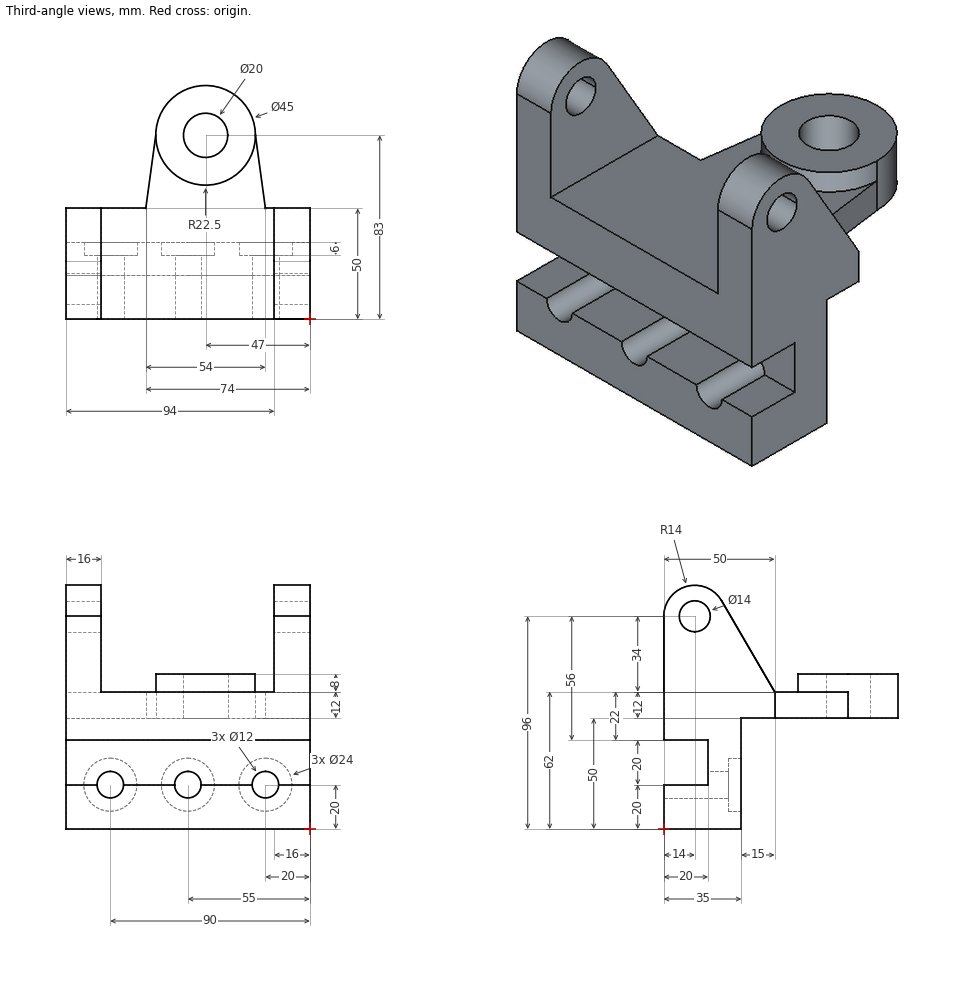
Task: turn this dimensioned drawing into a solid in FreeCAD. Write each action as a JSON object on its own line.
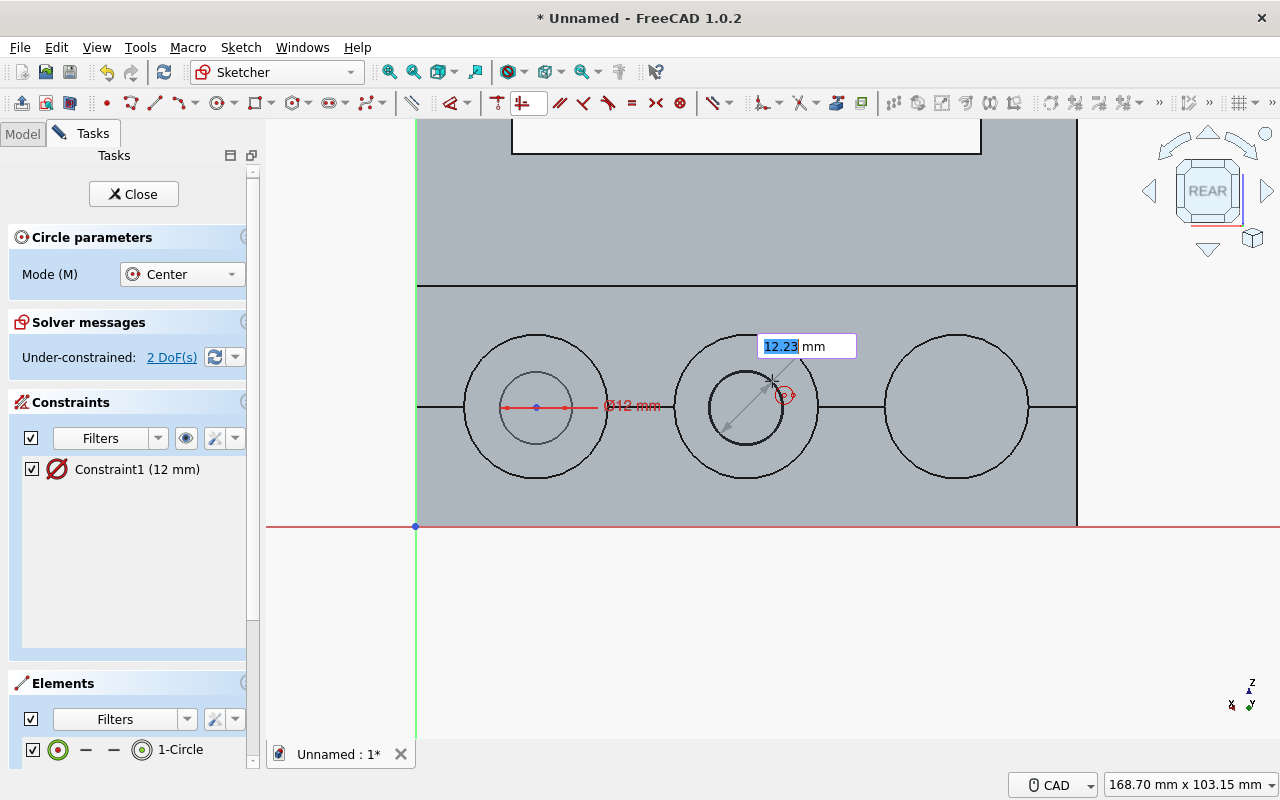
{"action": "type", "text": "12"}
{"action": "key", "text": "Return"}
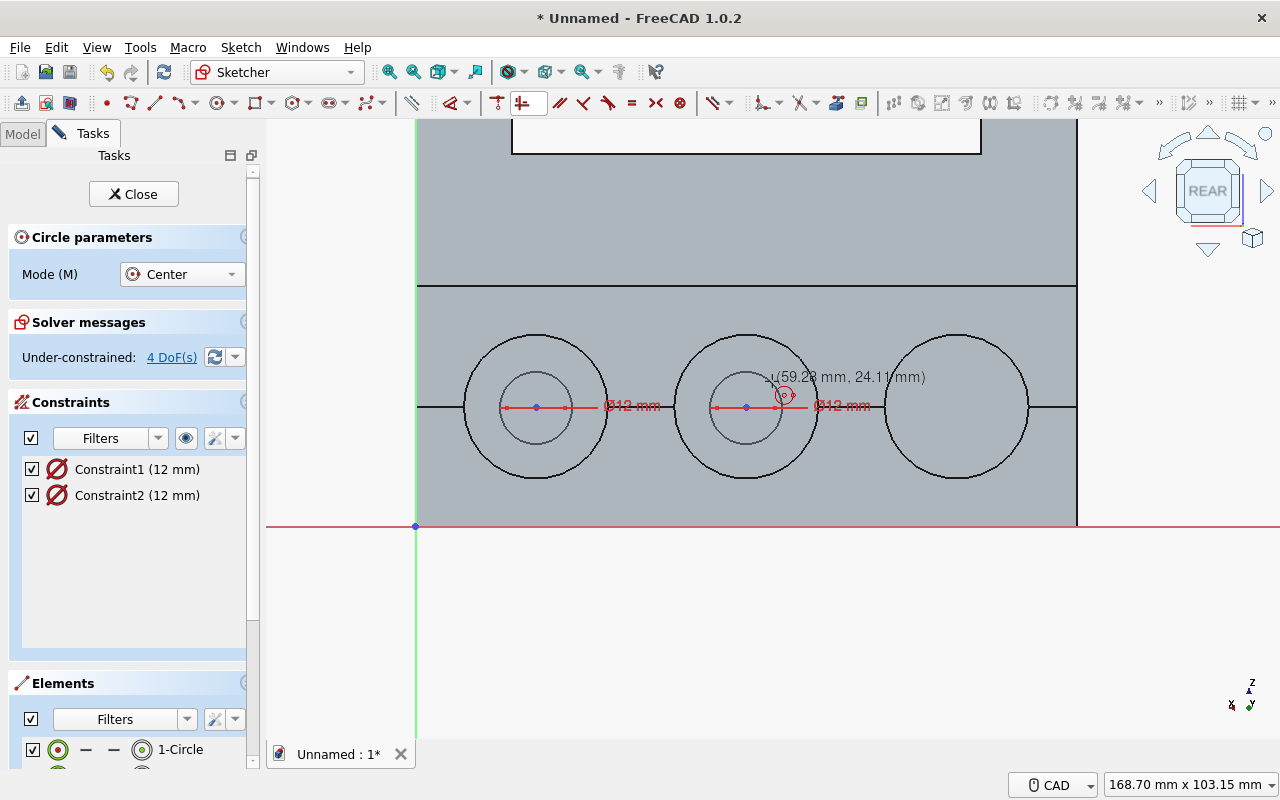
{"action": "left_click", "coordinate": [957, 407]}
{"action": "mouse_move", "coordinate": [982, 381]}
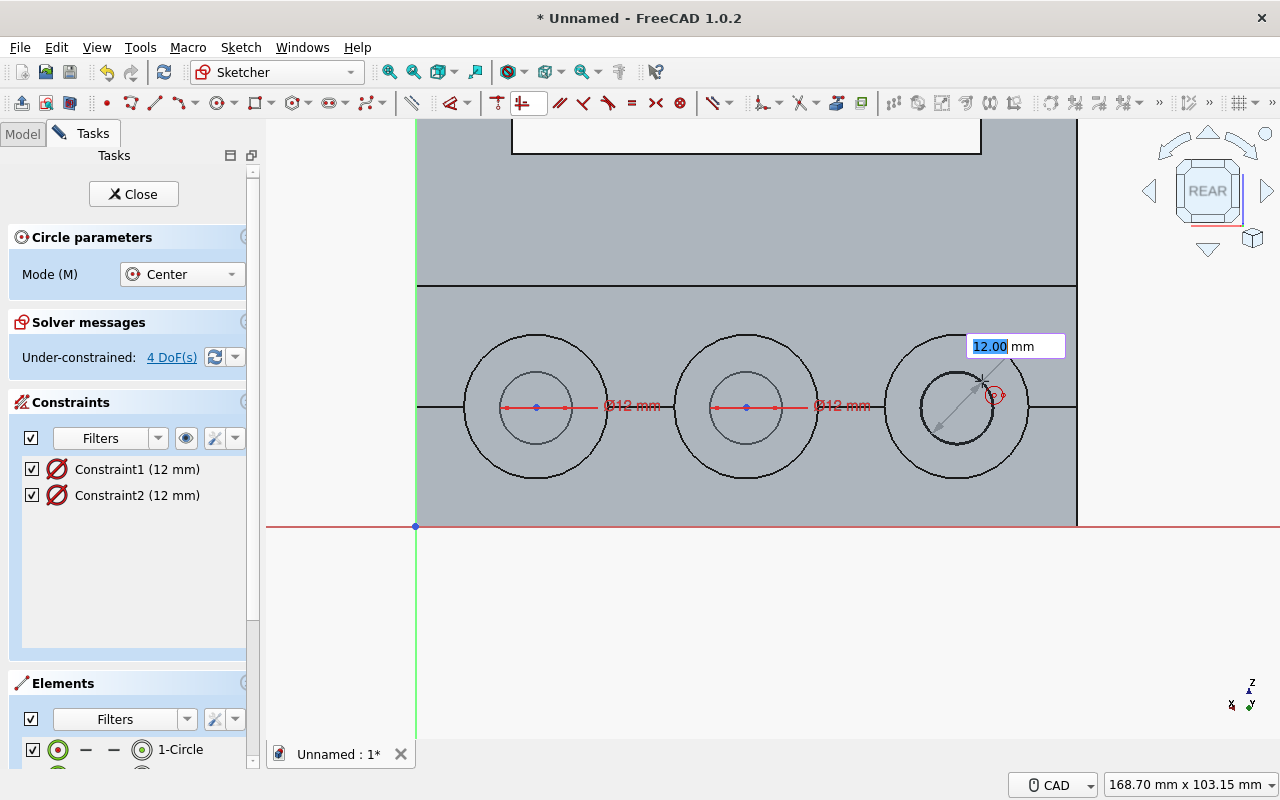
{"action": "type", "text": "12"}
{"action": "key", "text": "Return"}
{"action": "key", "text": "Escape"}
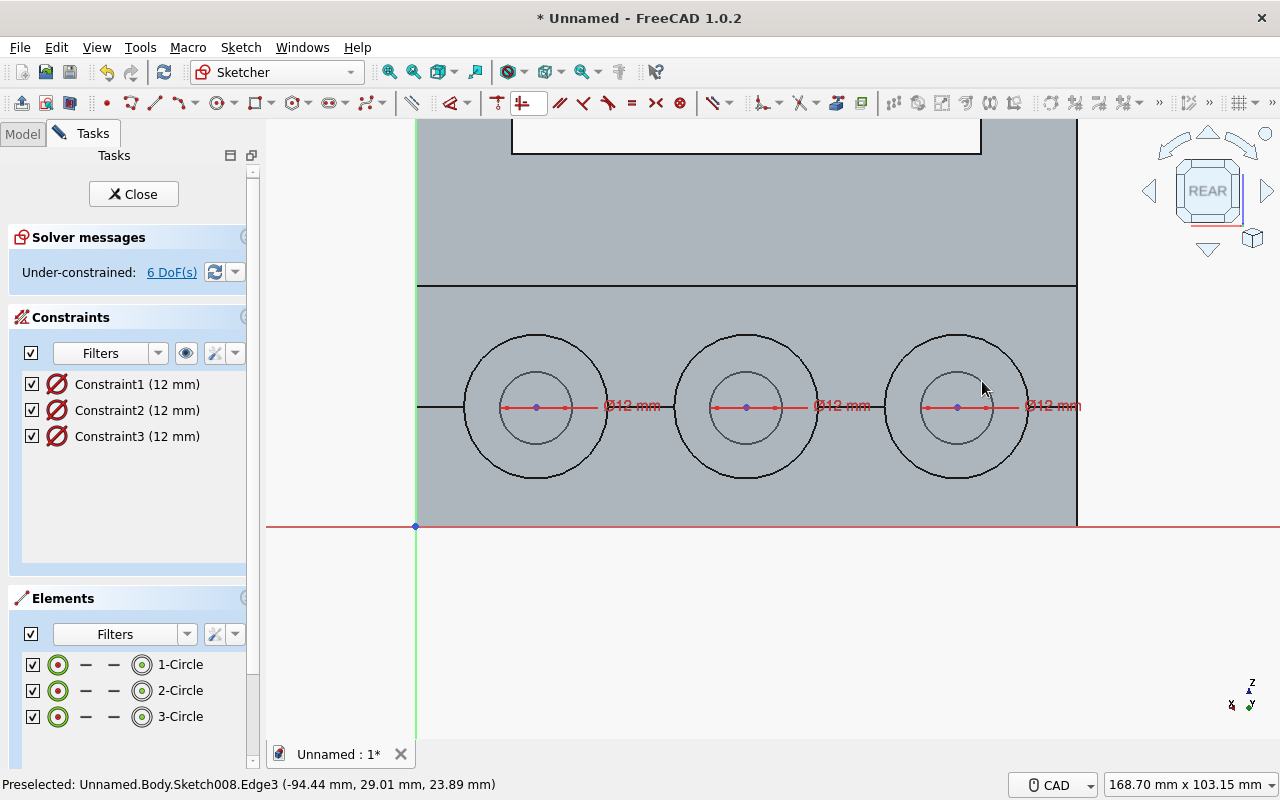
{"action": "left_click", "coordinate": [536, 408]}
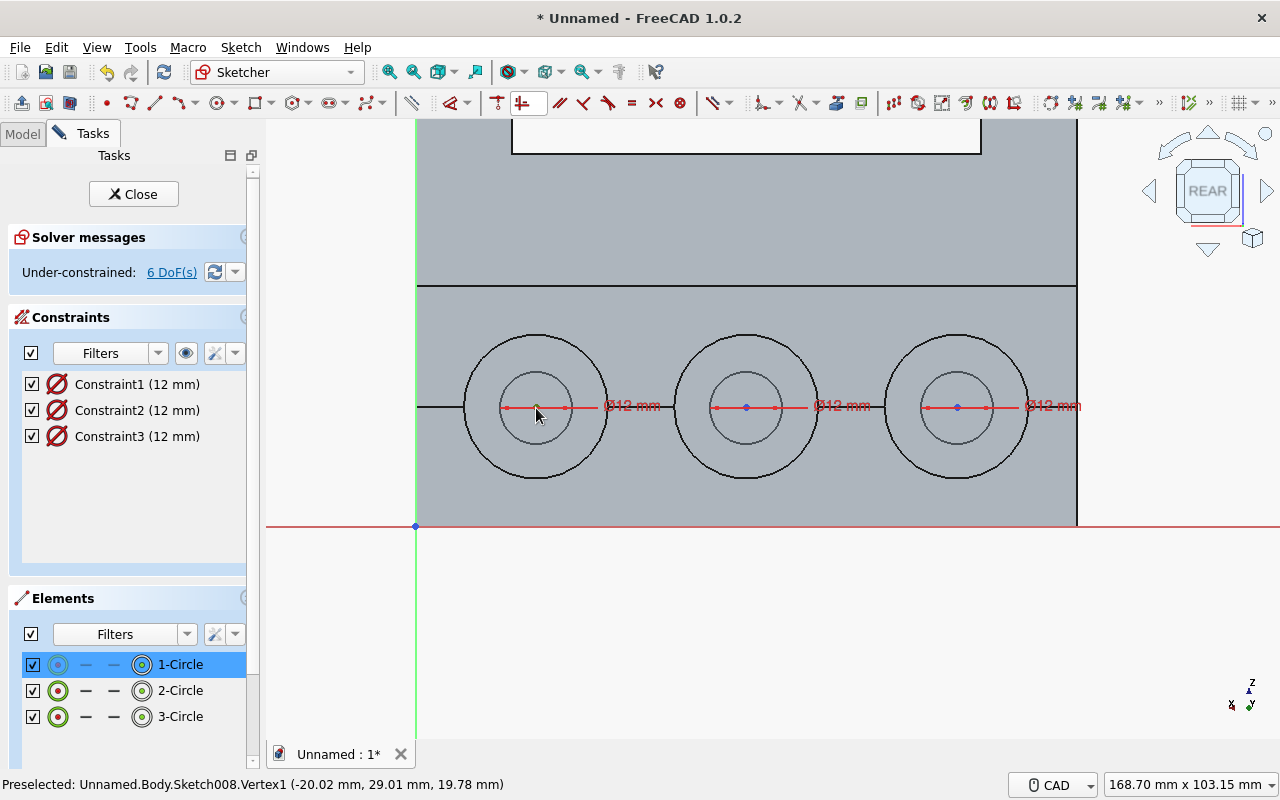
{"action": "left_click", "coordinate": [746, 408]}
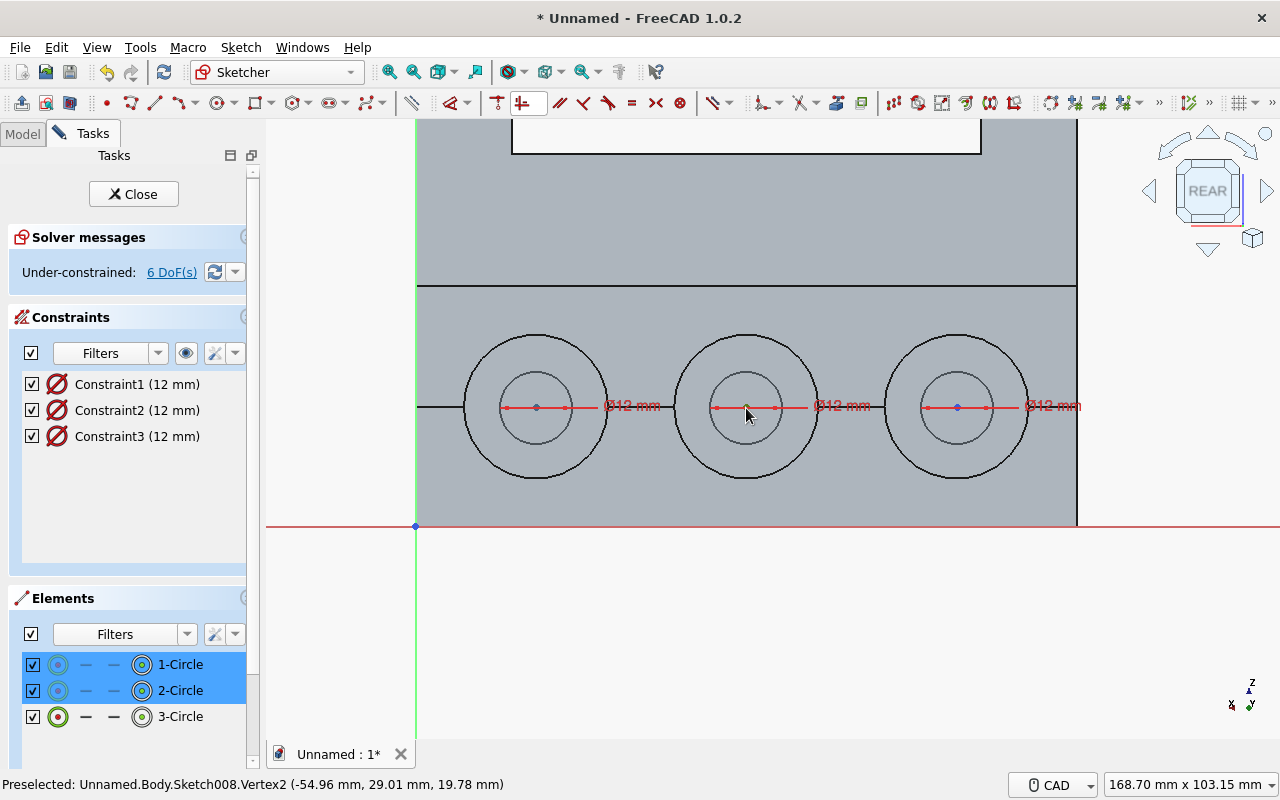
{"action": "left_click", "coordinate": [542, 104]}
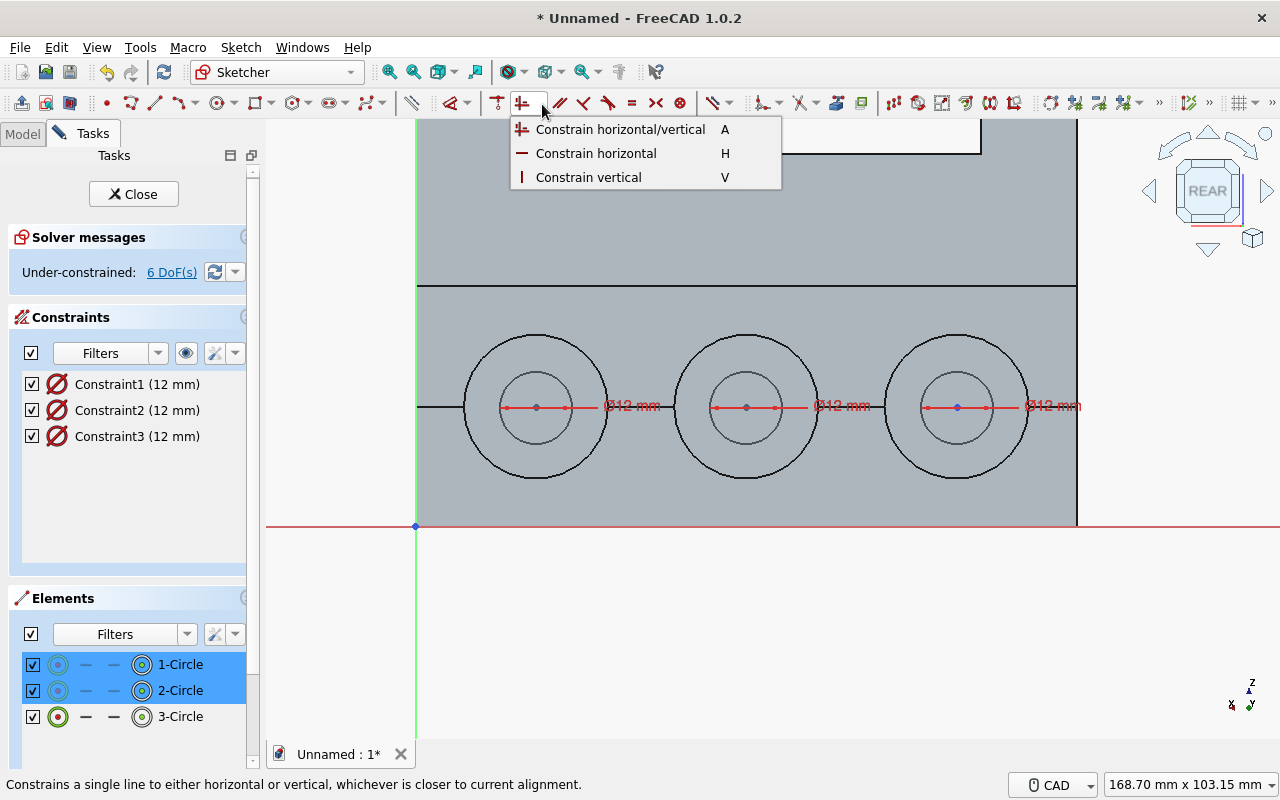
{"action": "left_click", "coordinate": [646, 153]}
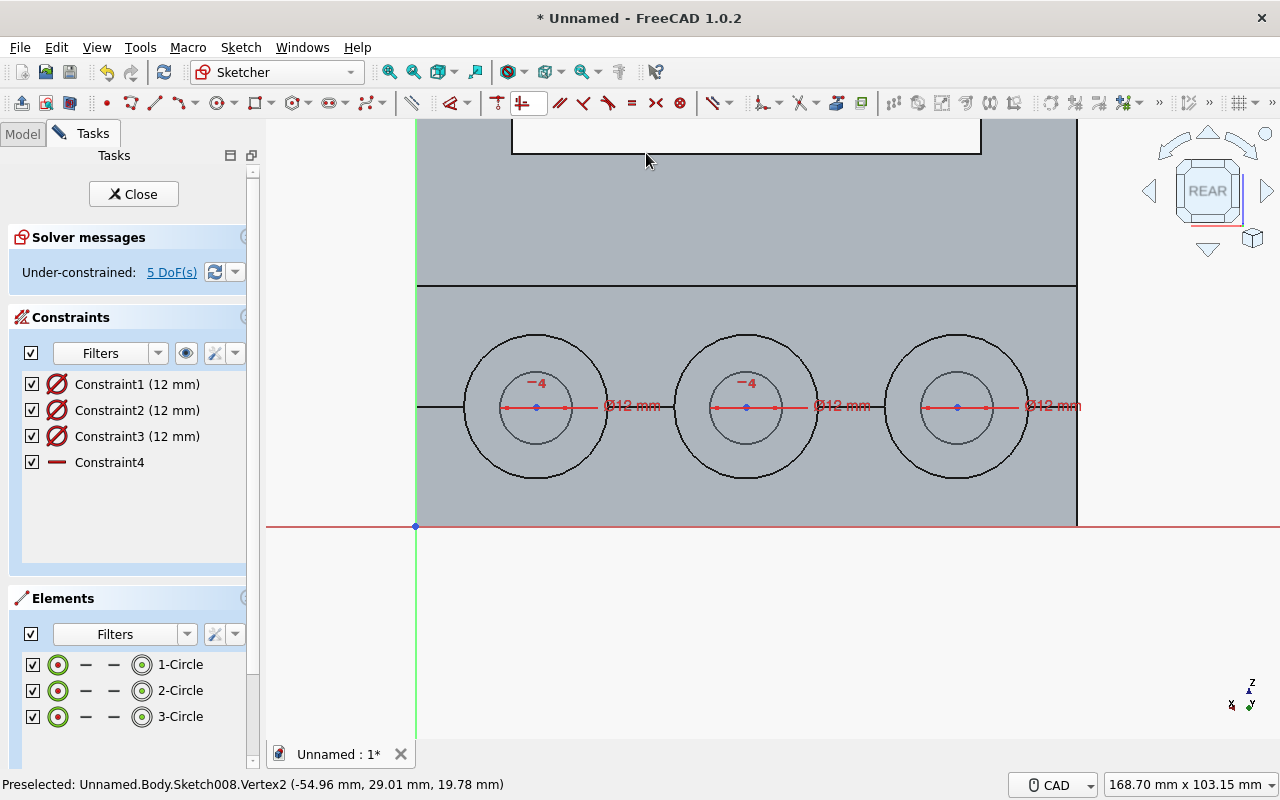
{"action": "left_click", "coordinate": [746, 408]}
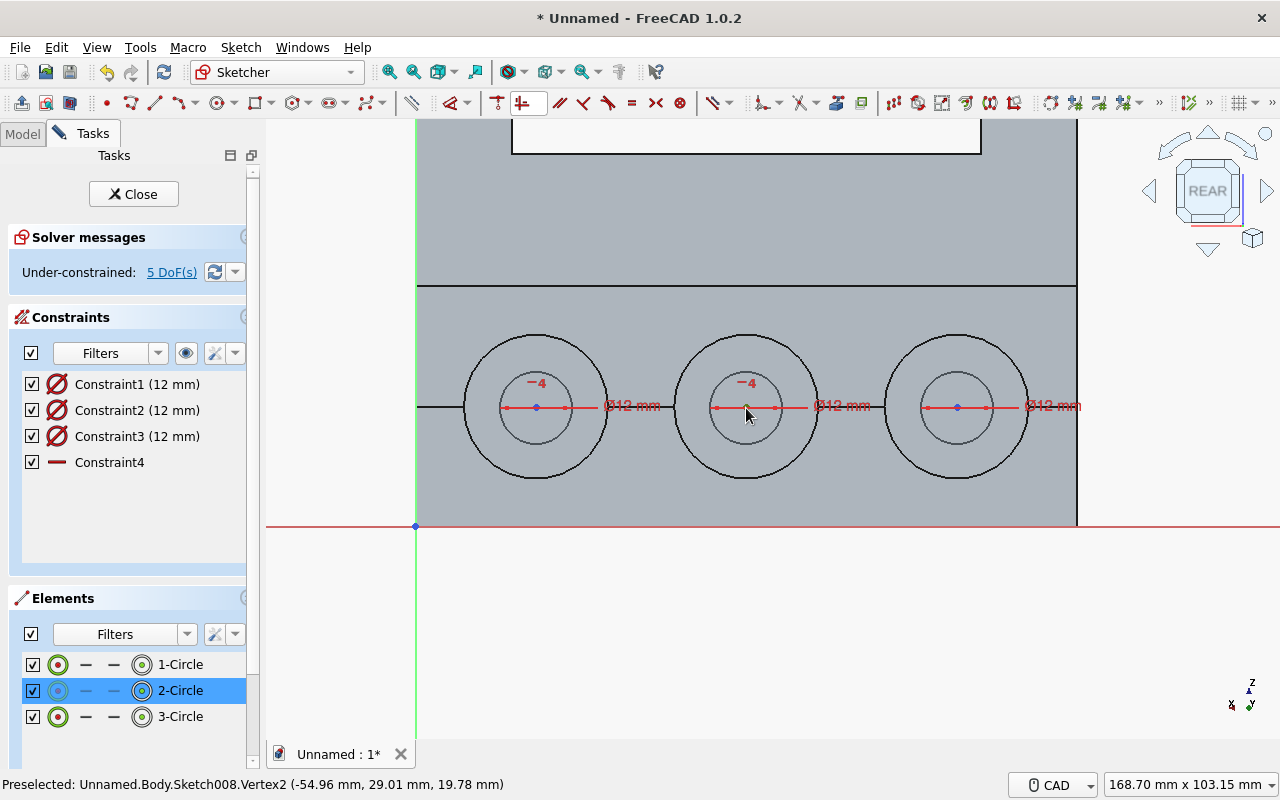
{"action": "left_click", "coordinate": [957, 408]}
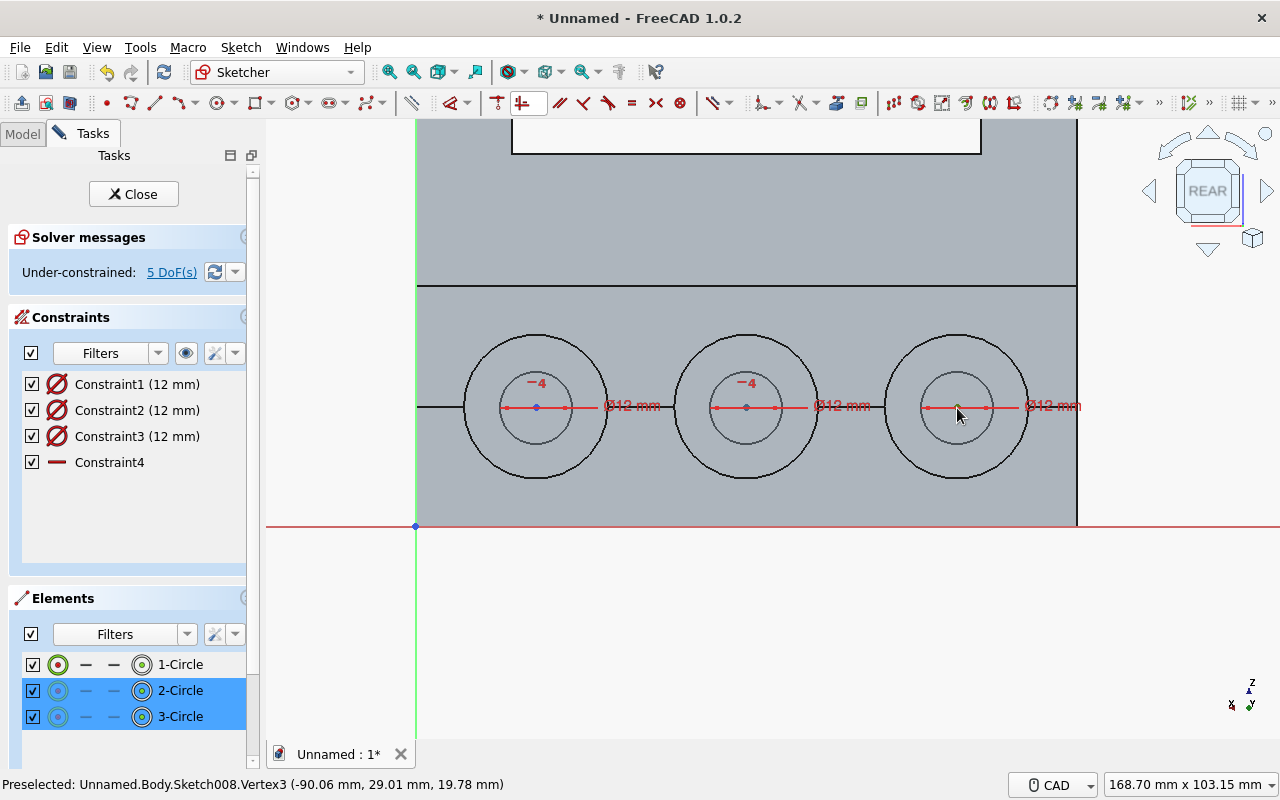
{"action": "key", "text": "h"}